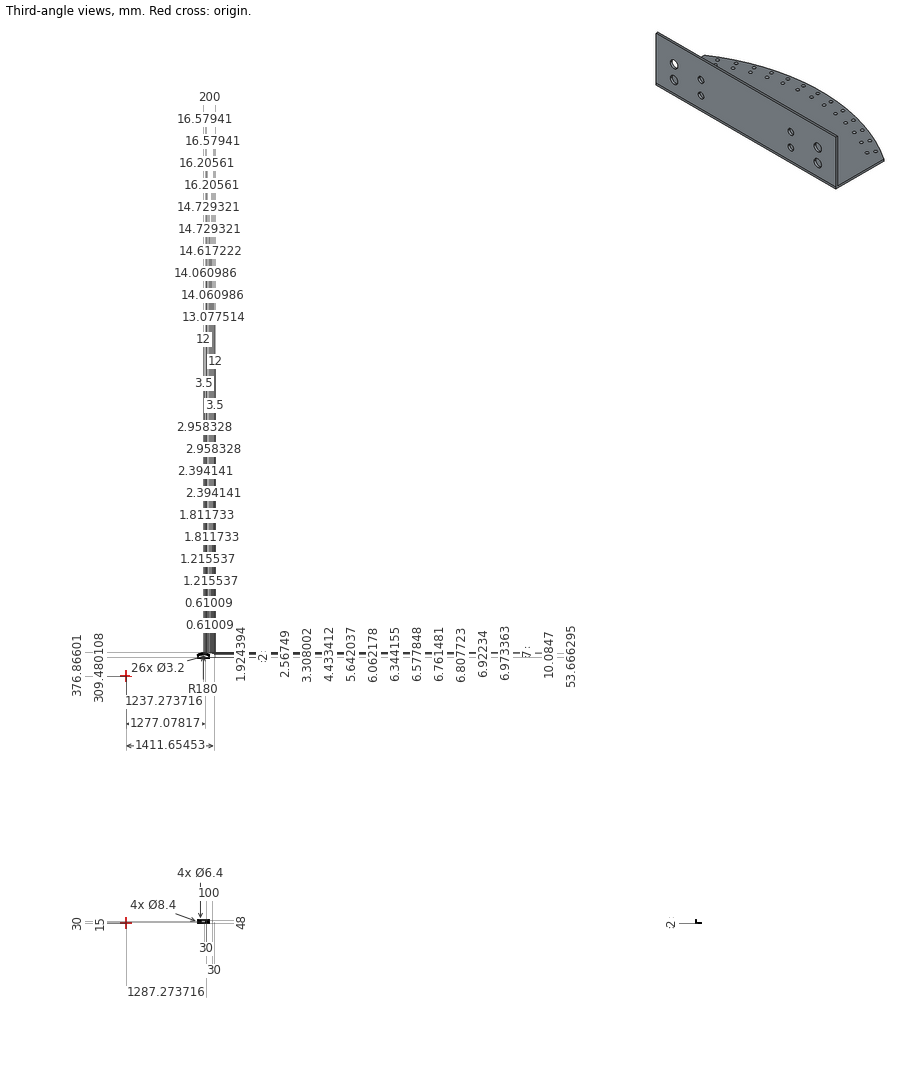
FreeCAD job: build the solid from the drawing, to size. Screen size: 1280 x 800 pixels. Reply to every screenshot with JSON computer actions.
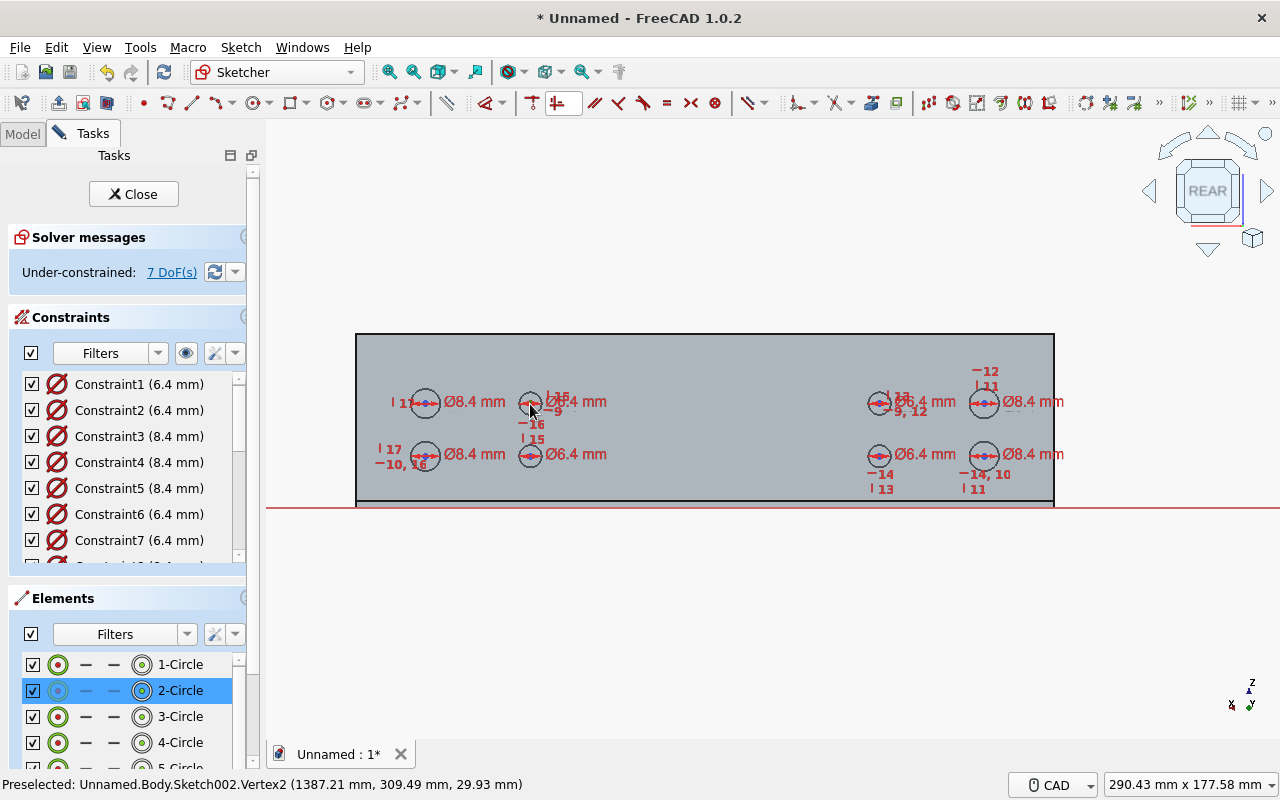
{"action": "left_click", "coordinate": [426, 404]}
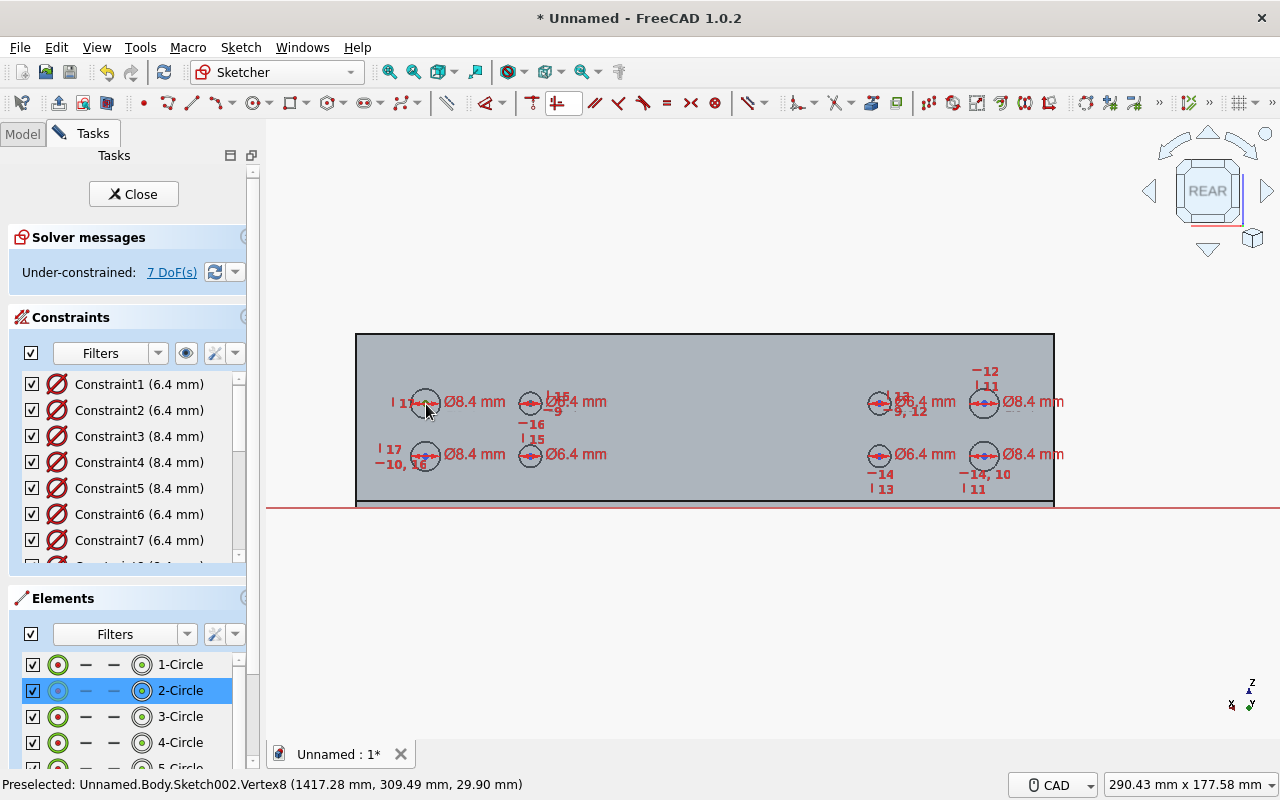
{"action": "key", "text": "h"}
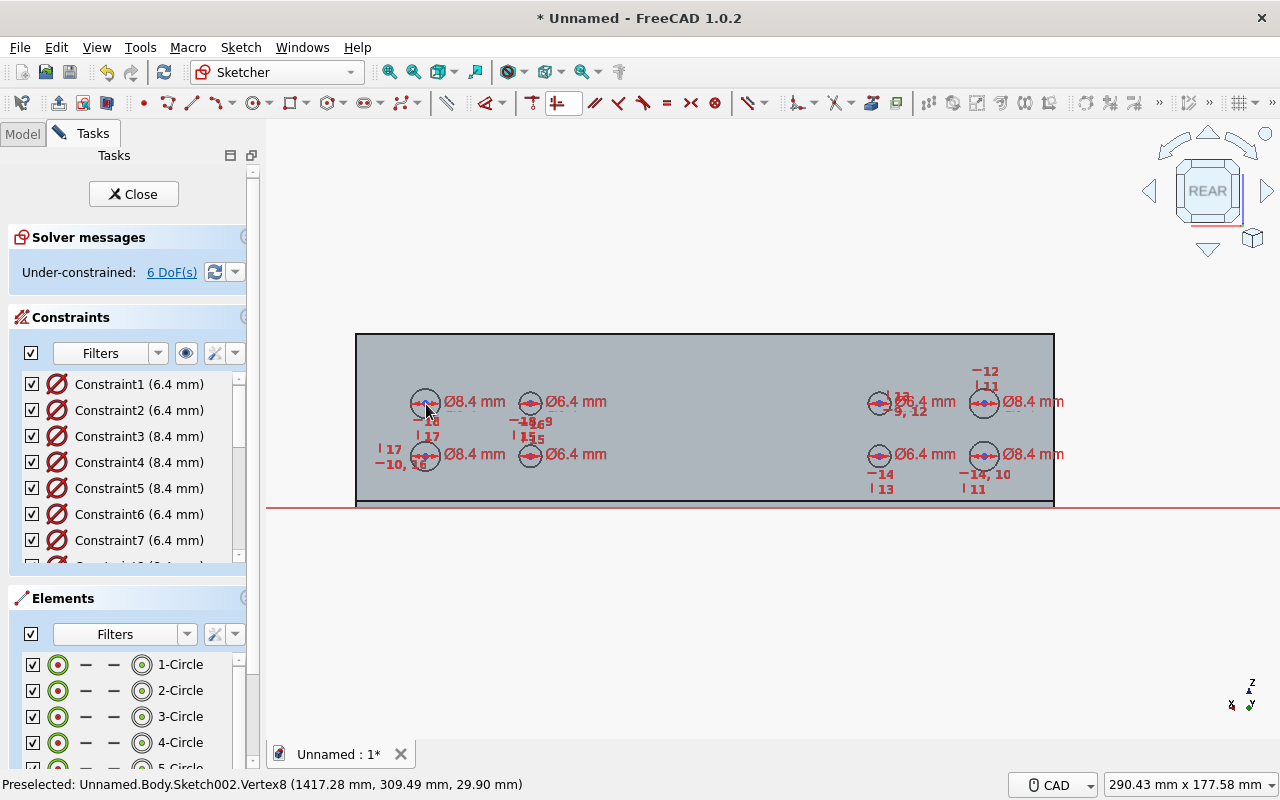
{"action": "key", "text": "d"}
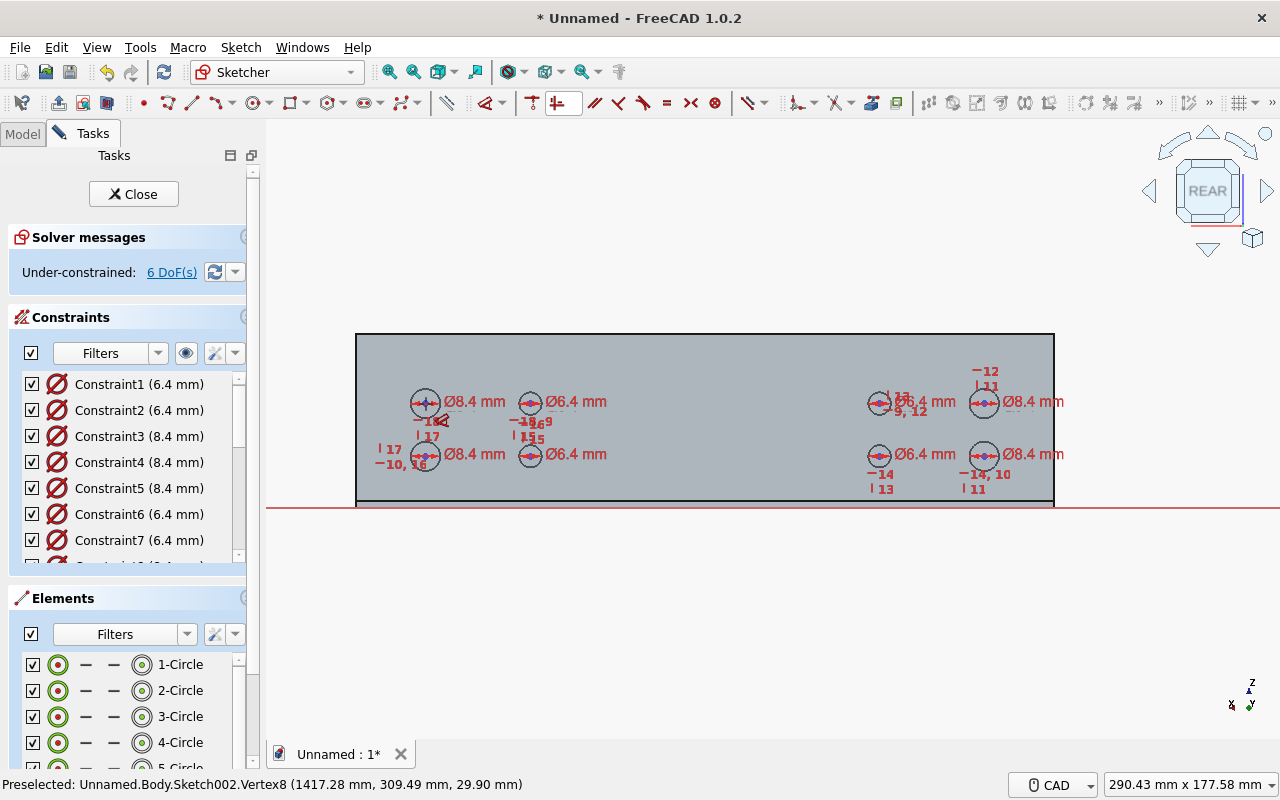
{"action": "left_click", "coordinate": [880, 404]}
{"action": "left_click", "coordinate": [846, 456]}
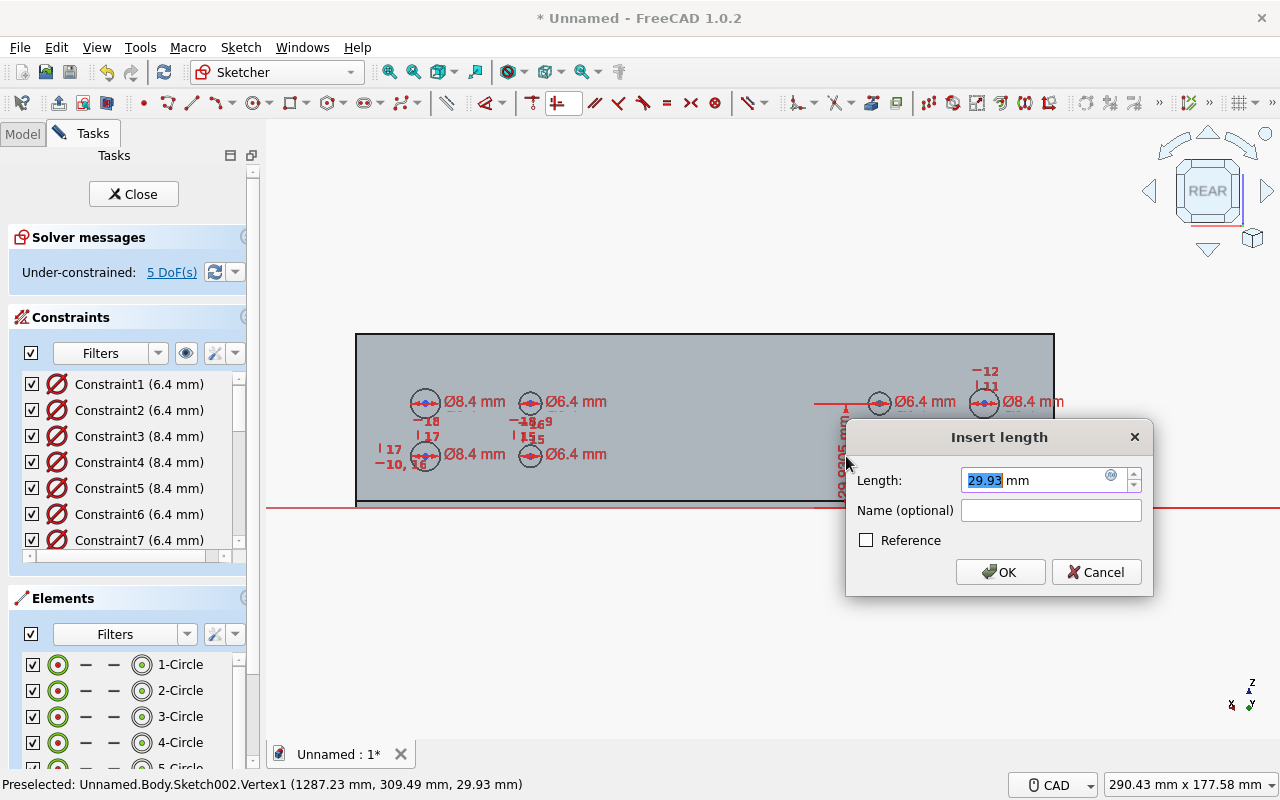
{"action": "type", "text": "30"}
{"action": "key", "text": "Return"}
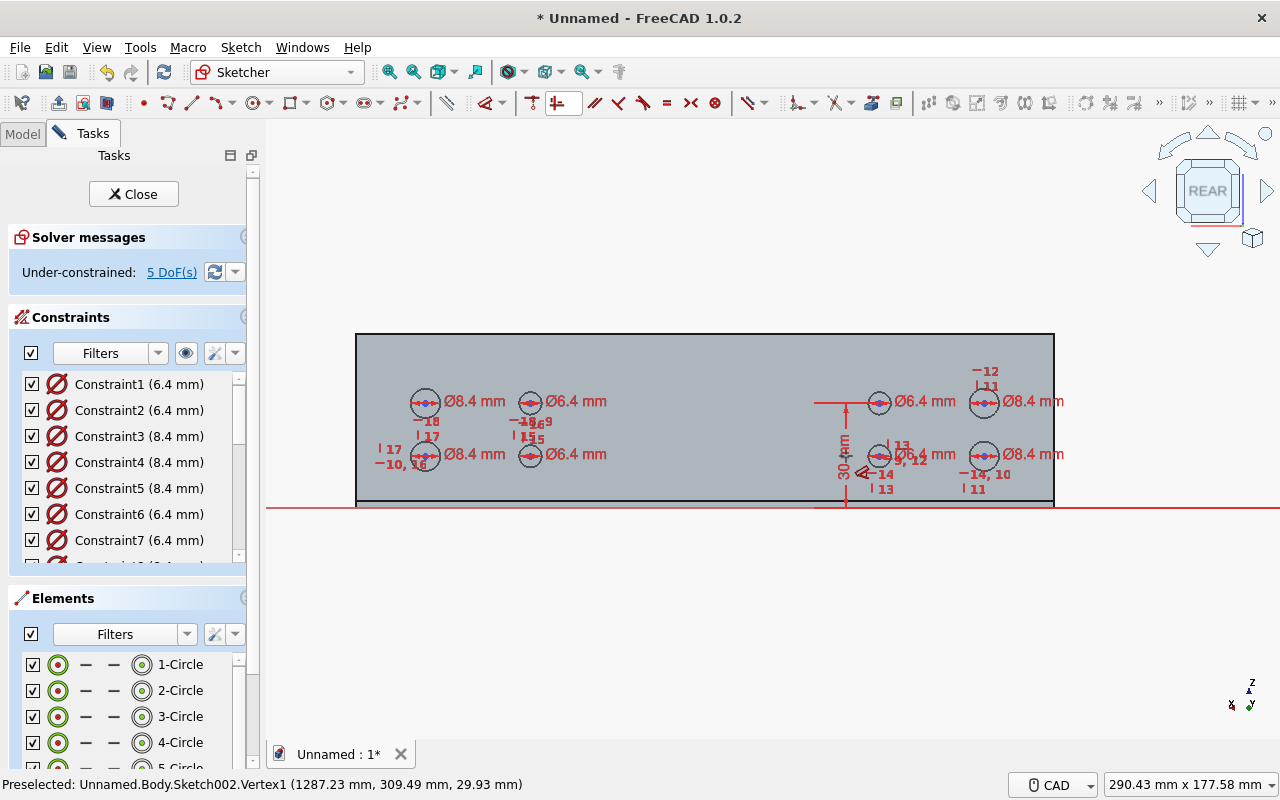
{"action": "left_click", "coordinate": [984, 456]}
{"action": "left_click", "coordinate": [950, 482]}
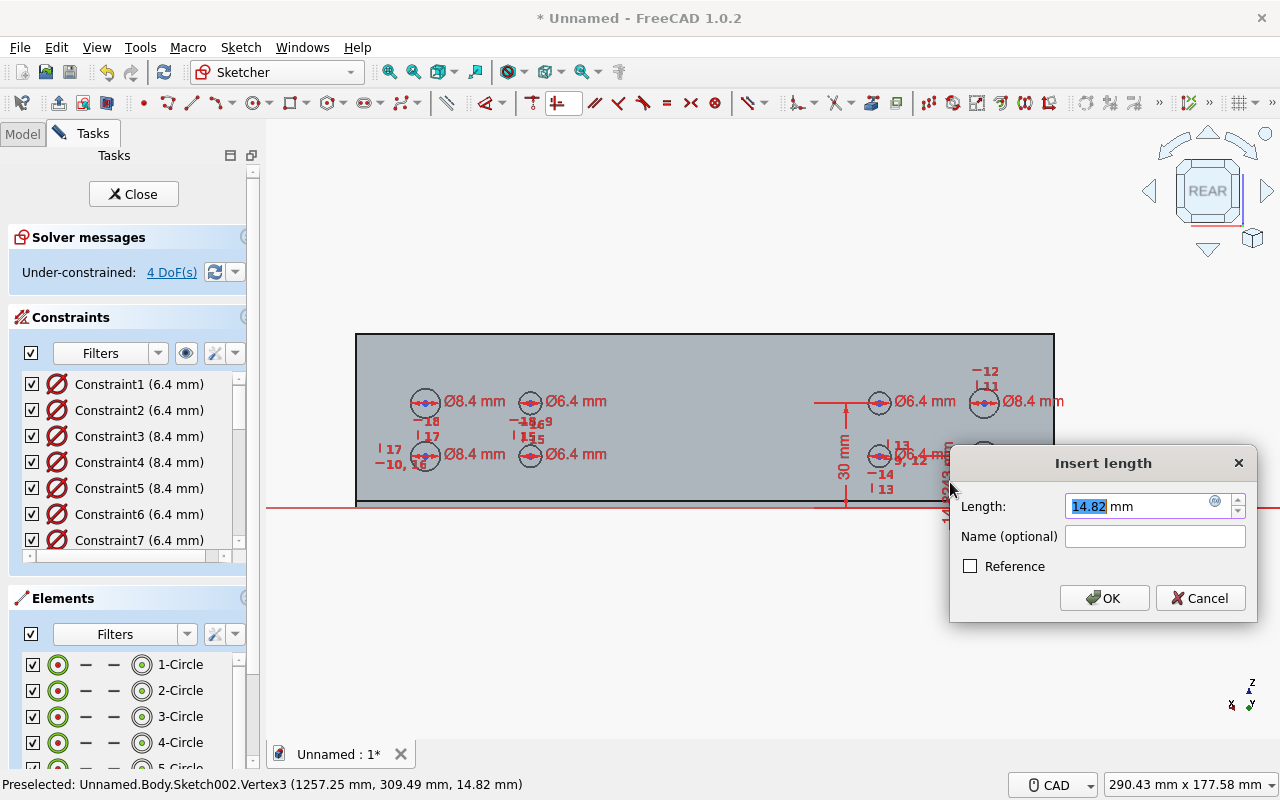
{"action": "type", "text": "15"}
{"action": "key", "text": "Return"}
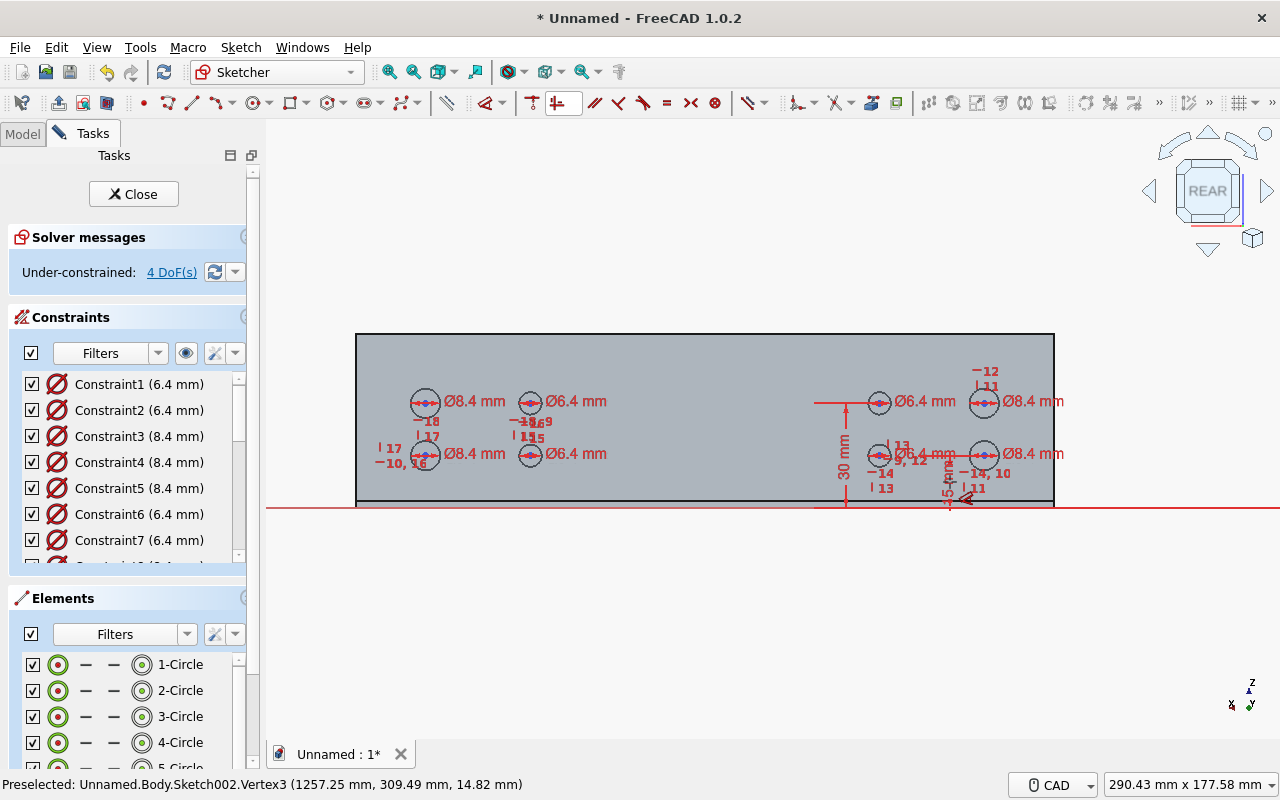
{"action": "left_click", "coordinate": [880, 403]}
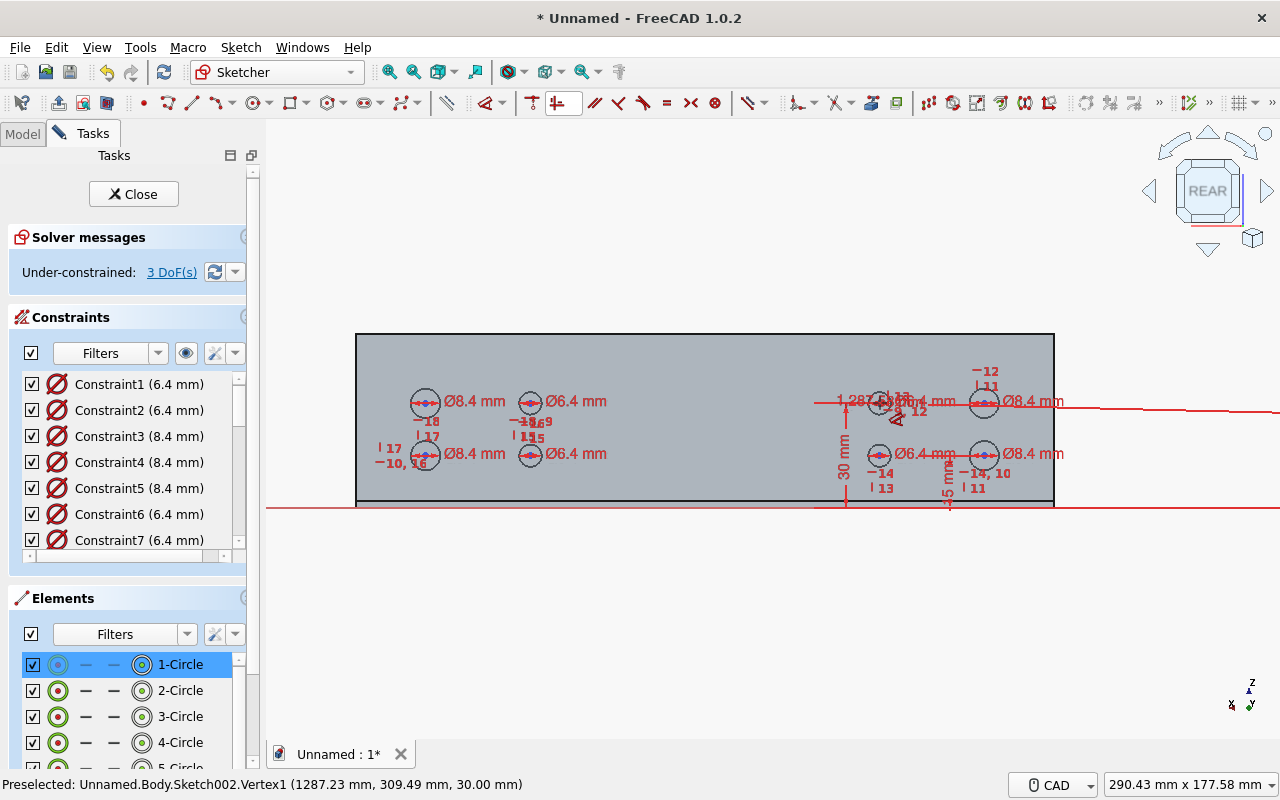
{"action": "left_click", "coordinate": [984, 456]}
{"action": "left_click", "coordinate": [932, 369]}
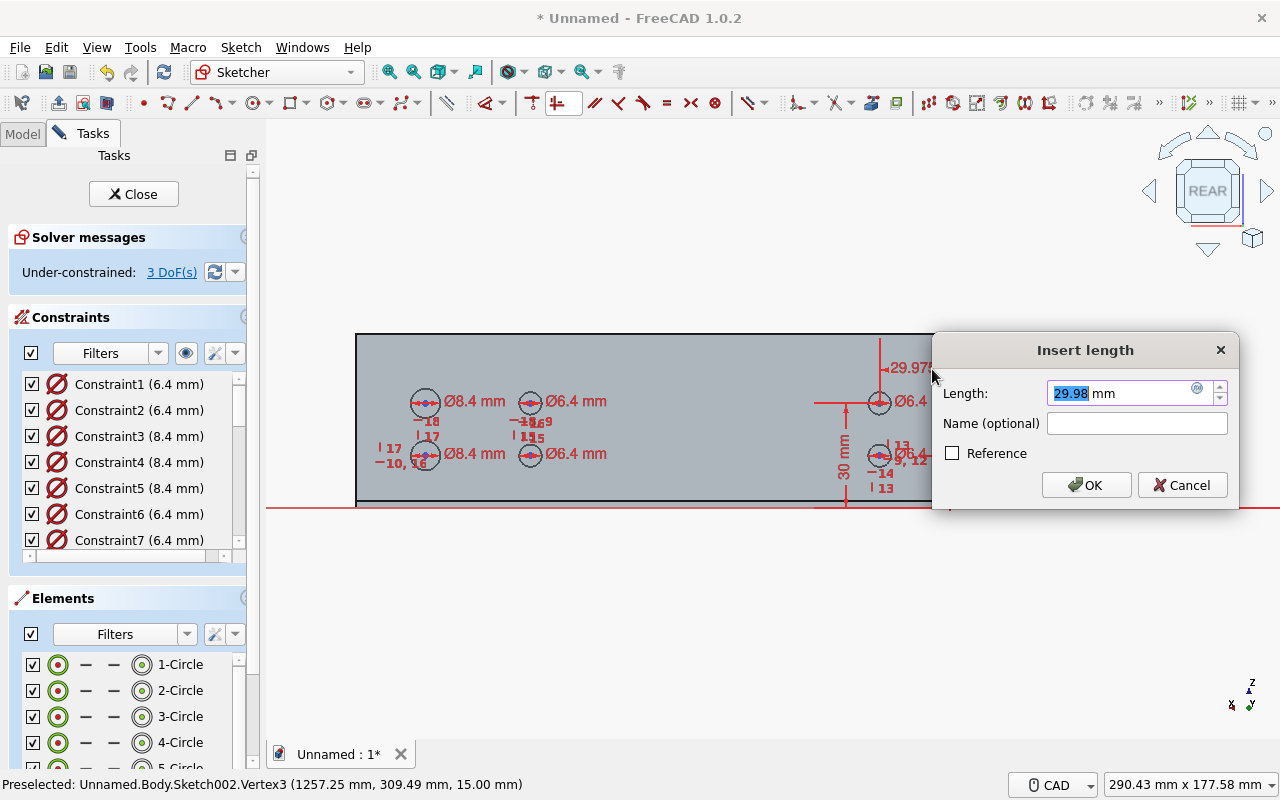
{"action": "type", "text": "30"}
{"action": "key", "text": "Return"}